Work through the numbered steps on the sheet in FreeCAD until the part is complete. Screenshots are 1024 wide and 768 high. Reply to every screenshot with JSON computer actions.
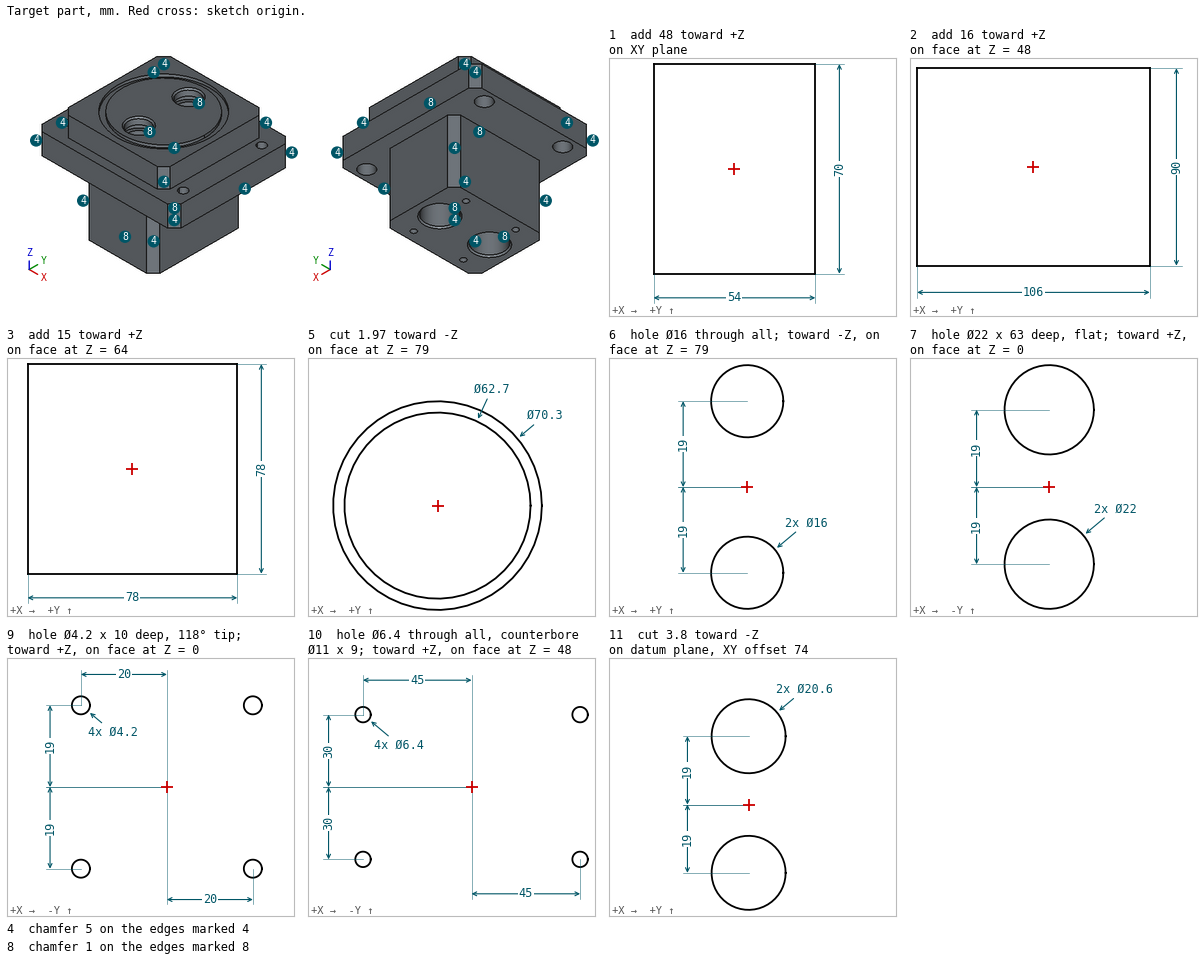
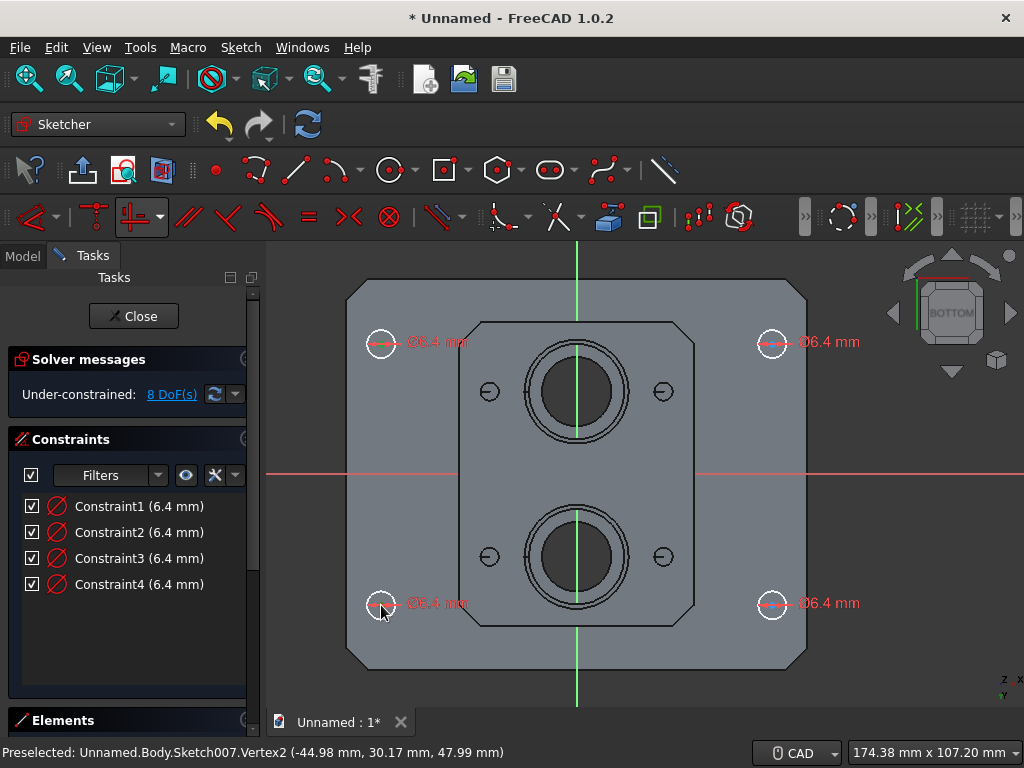
{"action": "left_click", "coordinate": [162, 218]}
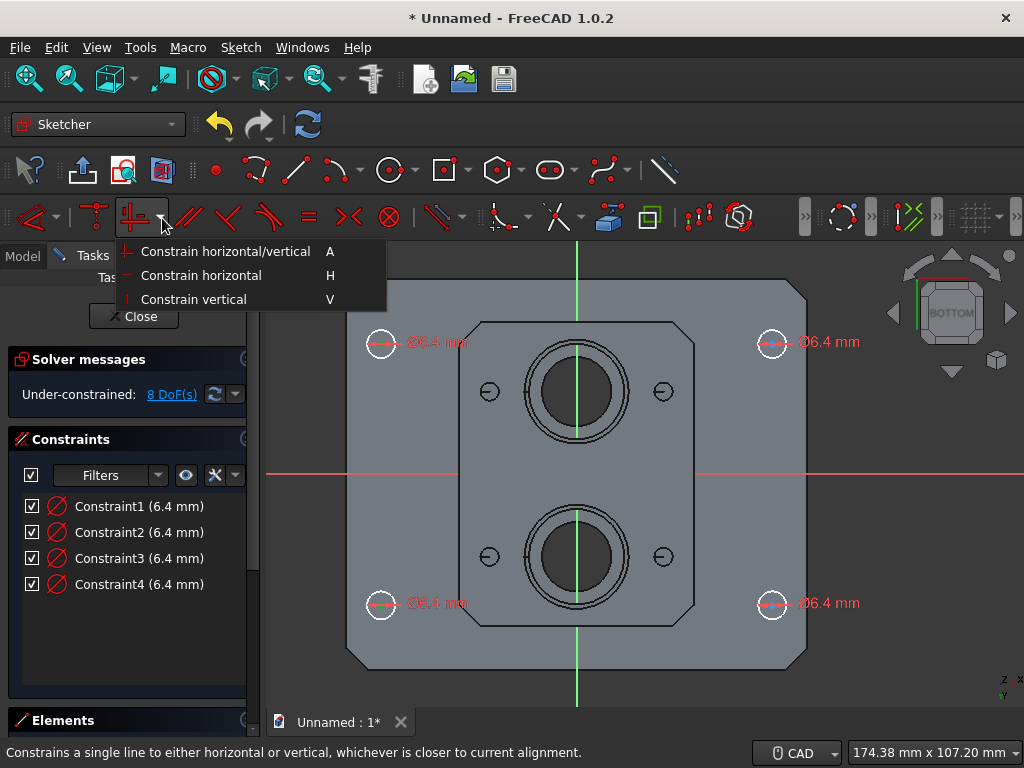
{"action": "left_click", "coordinate": [251, 299]}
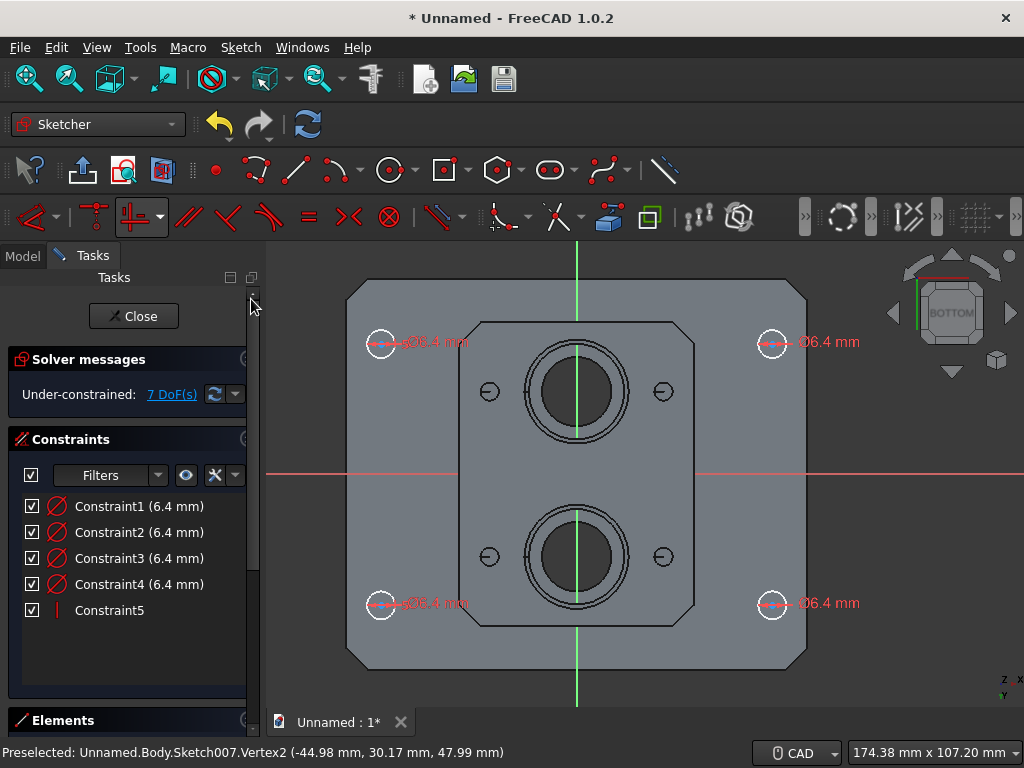
{"action": "left_click", "coordinate": [381, 605]}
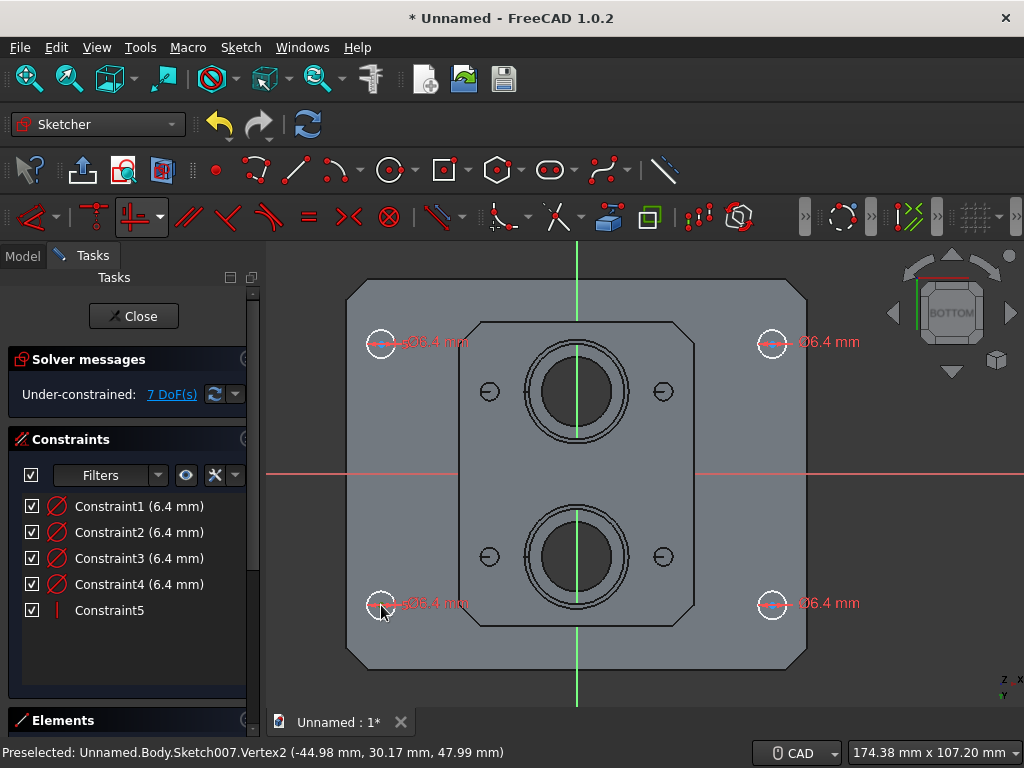
{"action": "left_click", "coordinate": [772, 605]}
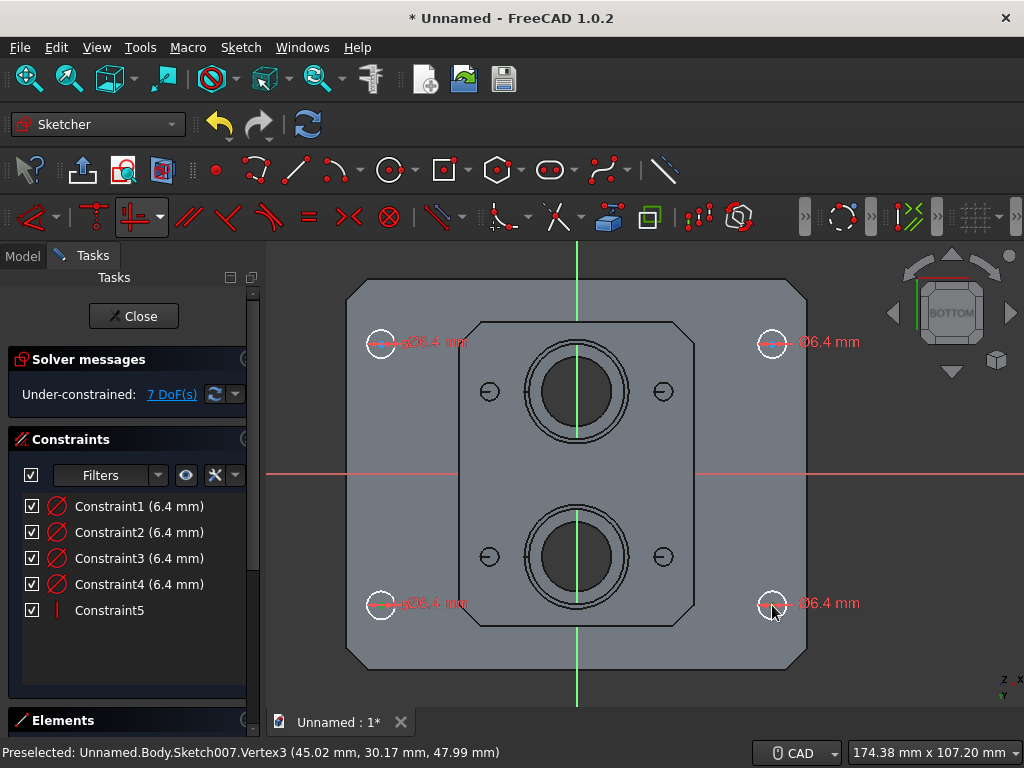
{"action": "left_click", "coordinate": [162, 218]}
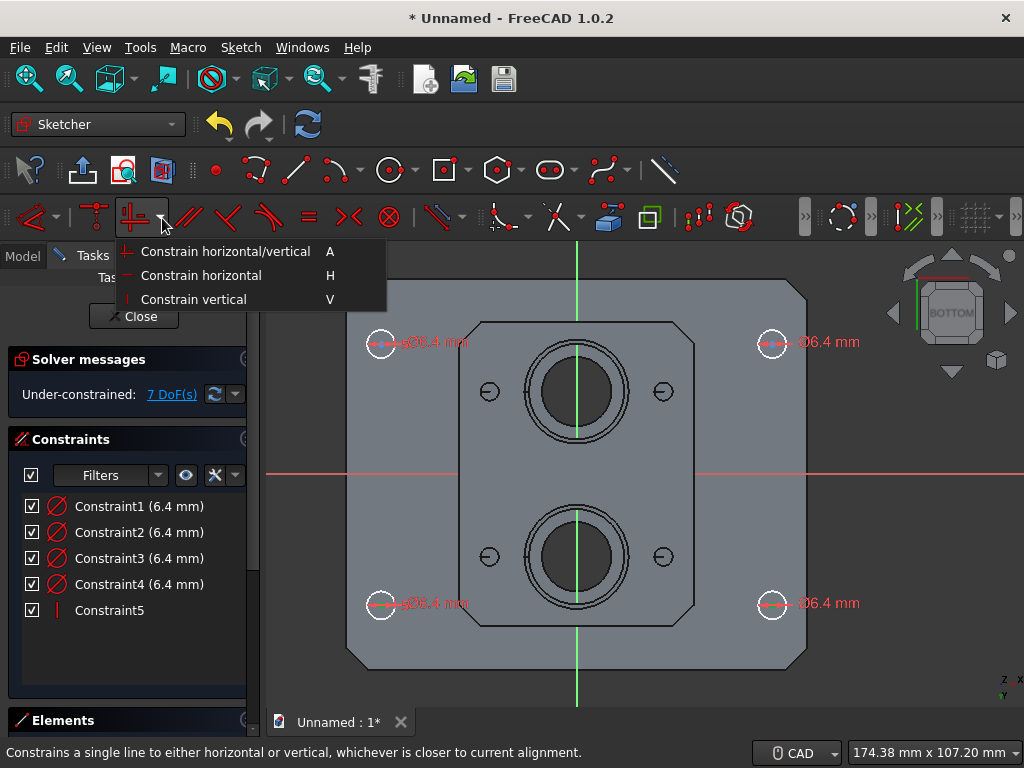
{"action": "left_click", "coordinate": [251, 275]}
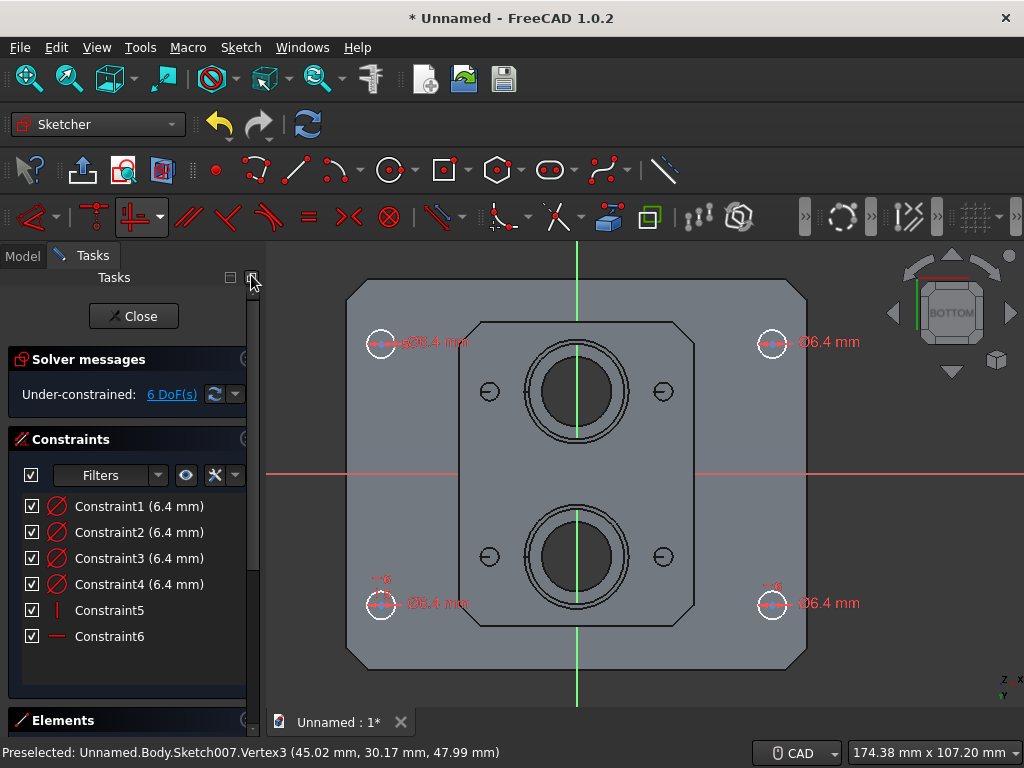
{"action": "left_click", "coordinate": [772, 605]}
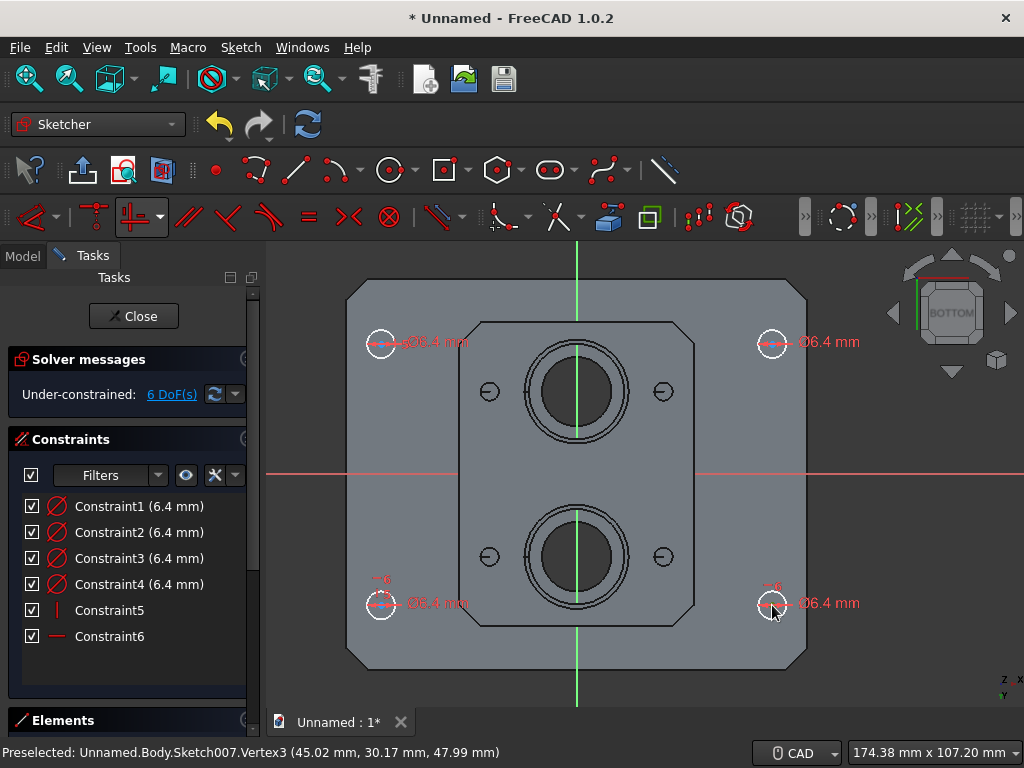
{"action": "left_click", "coordinate": [772, 344]}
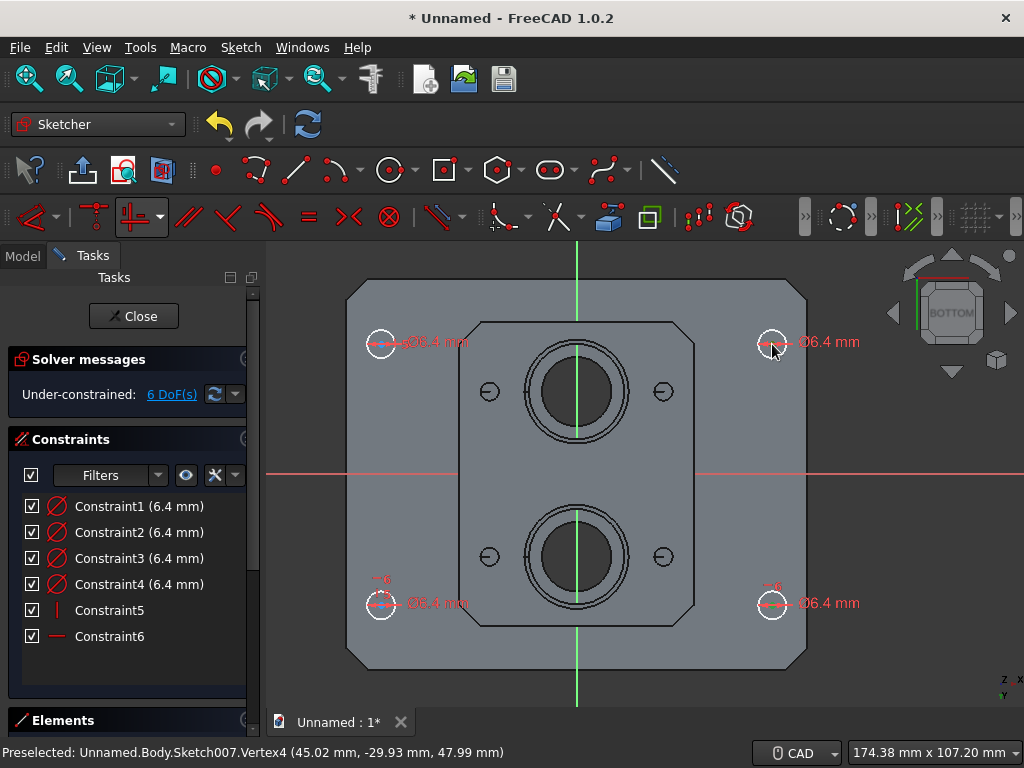
{"action": "key", "text": "v"}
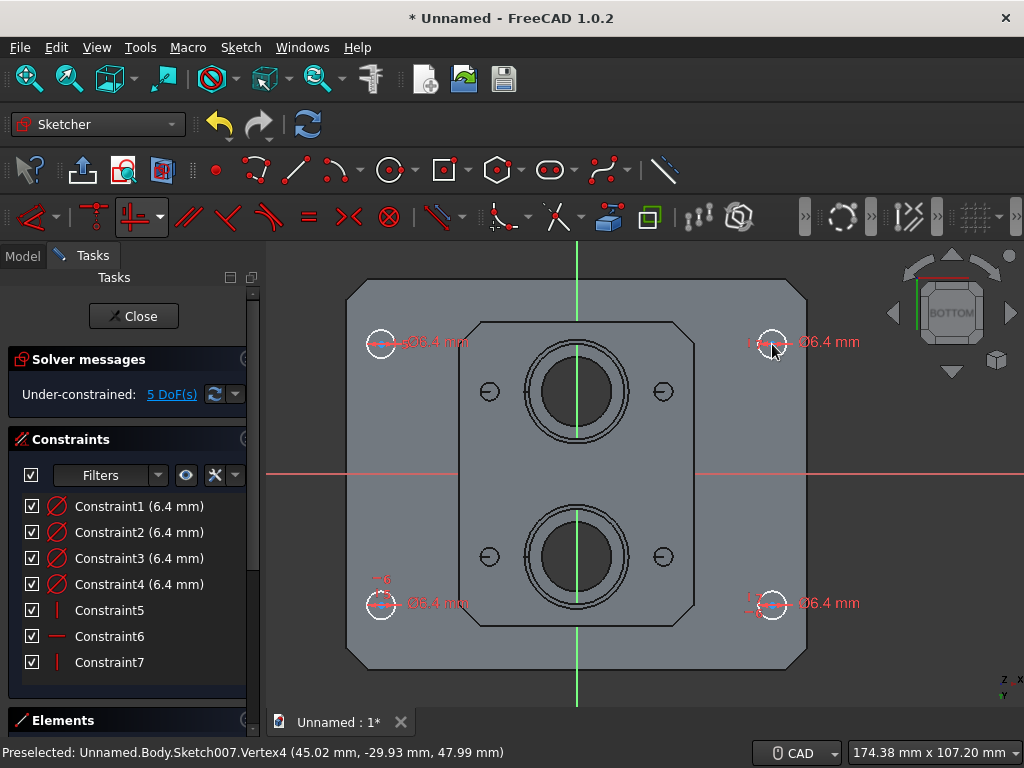
{"action": "left_click", "coordinate": [381, 344]}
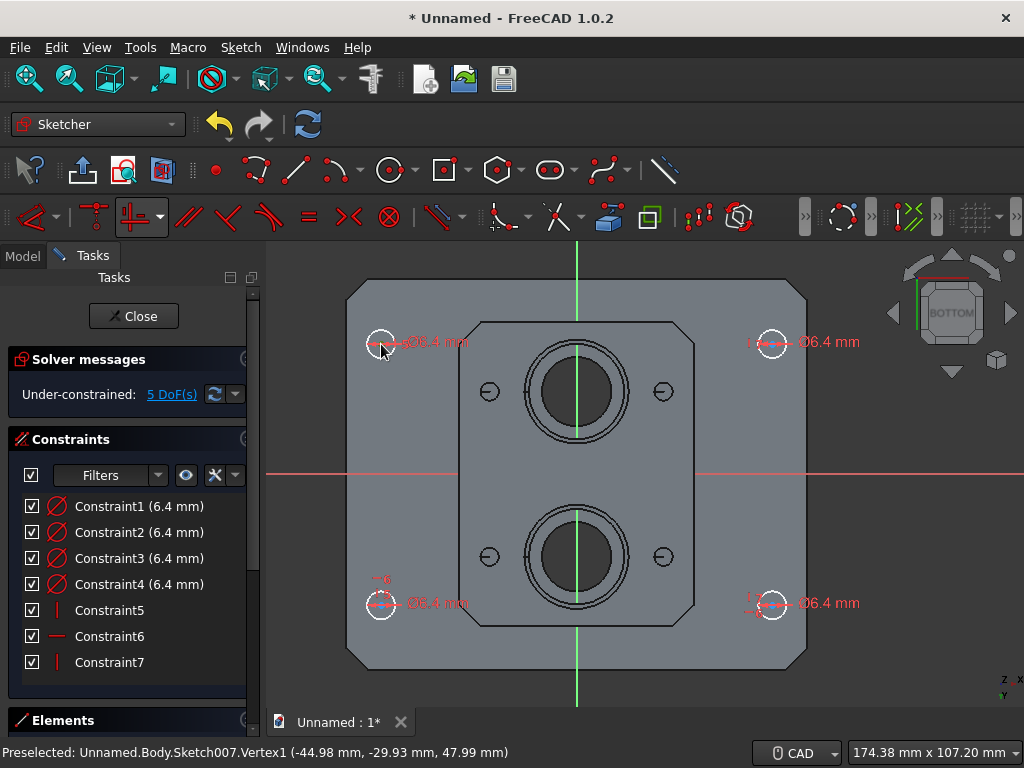
{"action": "left_click", "coordinate": [772, 344]}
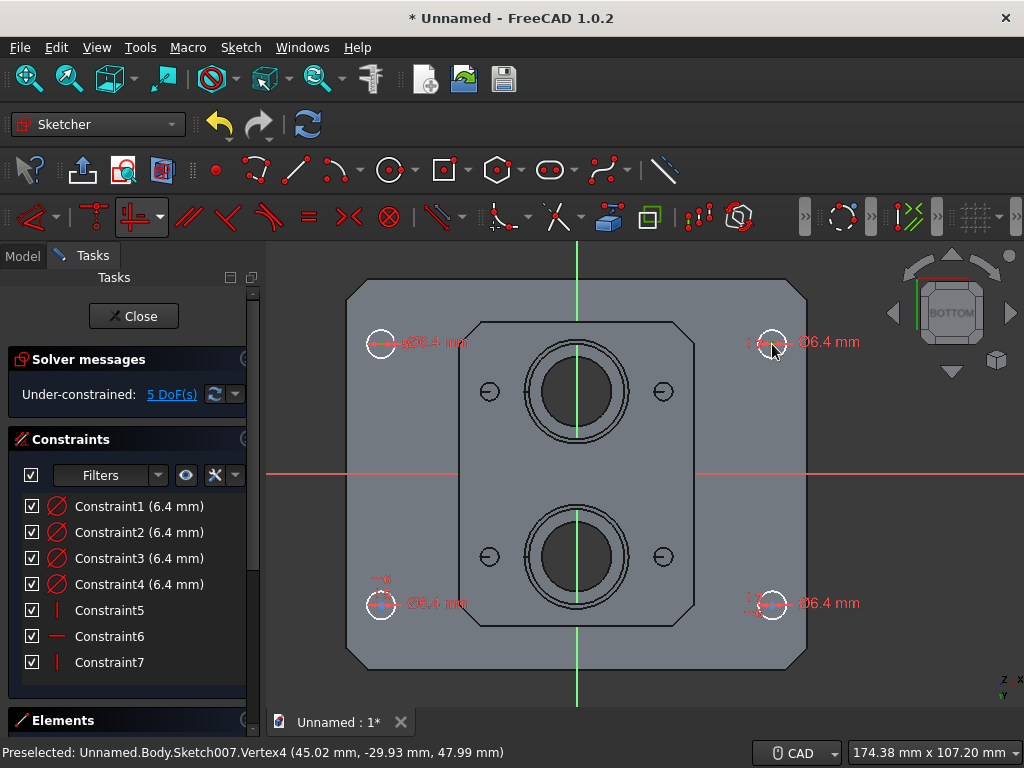
{"action": "key", "text": "h"}